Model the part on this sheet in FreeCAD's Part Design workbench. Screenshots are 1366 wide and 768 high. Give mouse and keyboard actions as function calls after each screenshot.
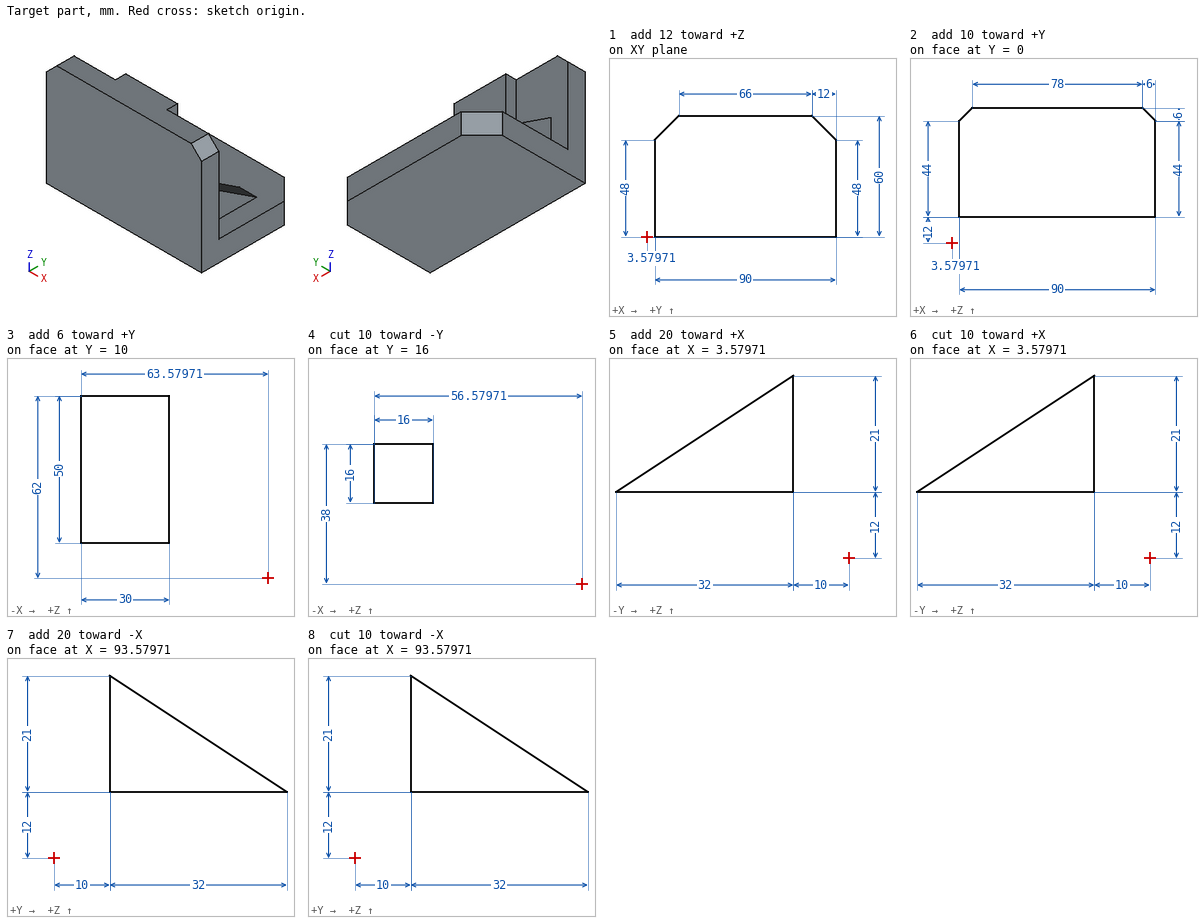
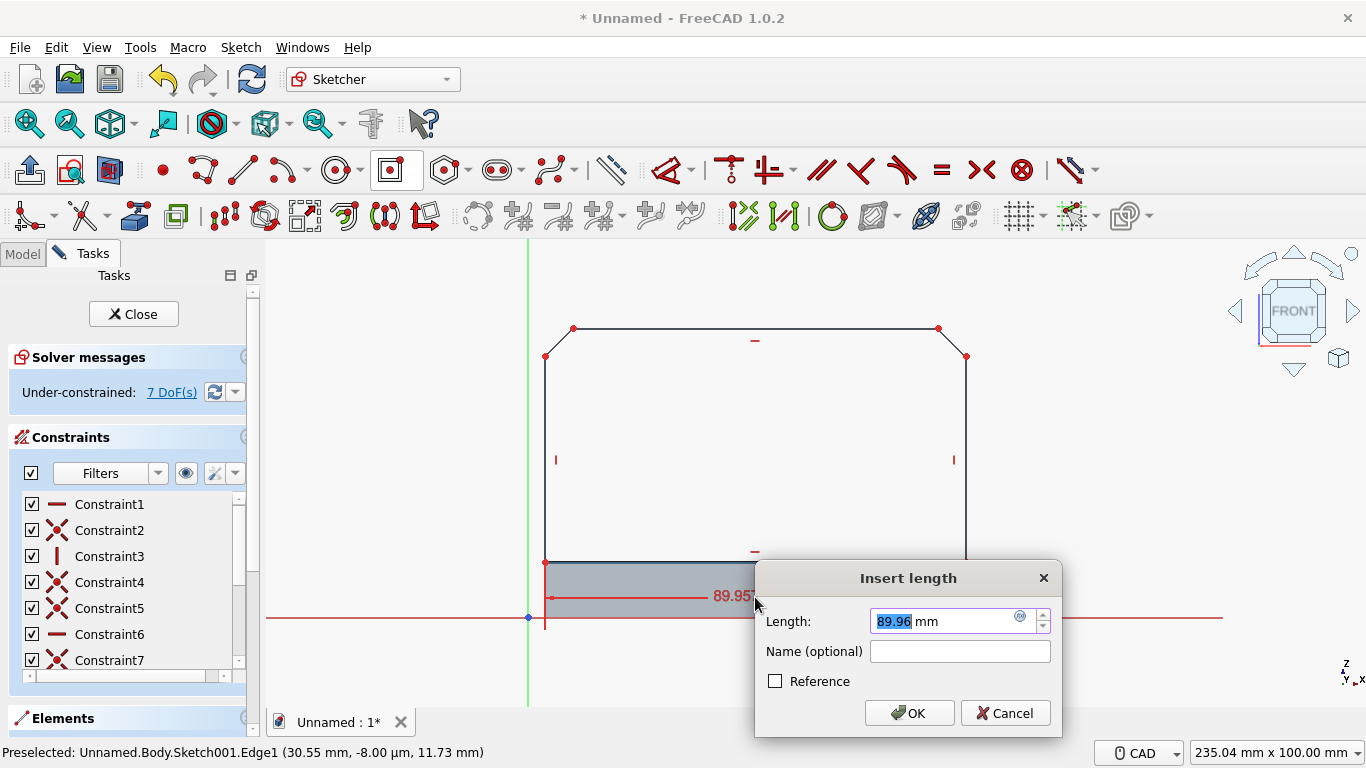
text(90)
key(Return)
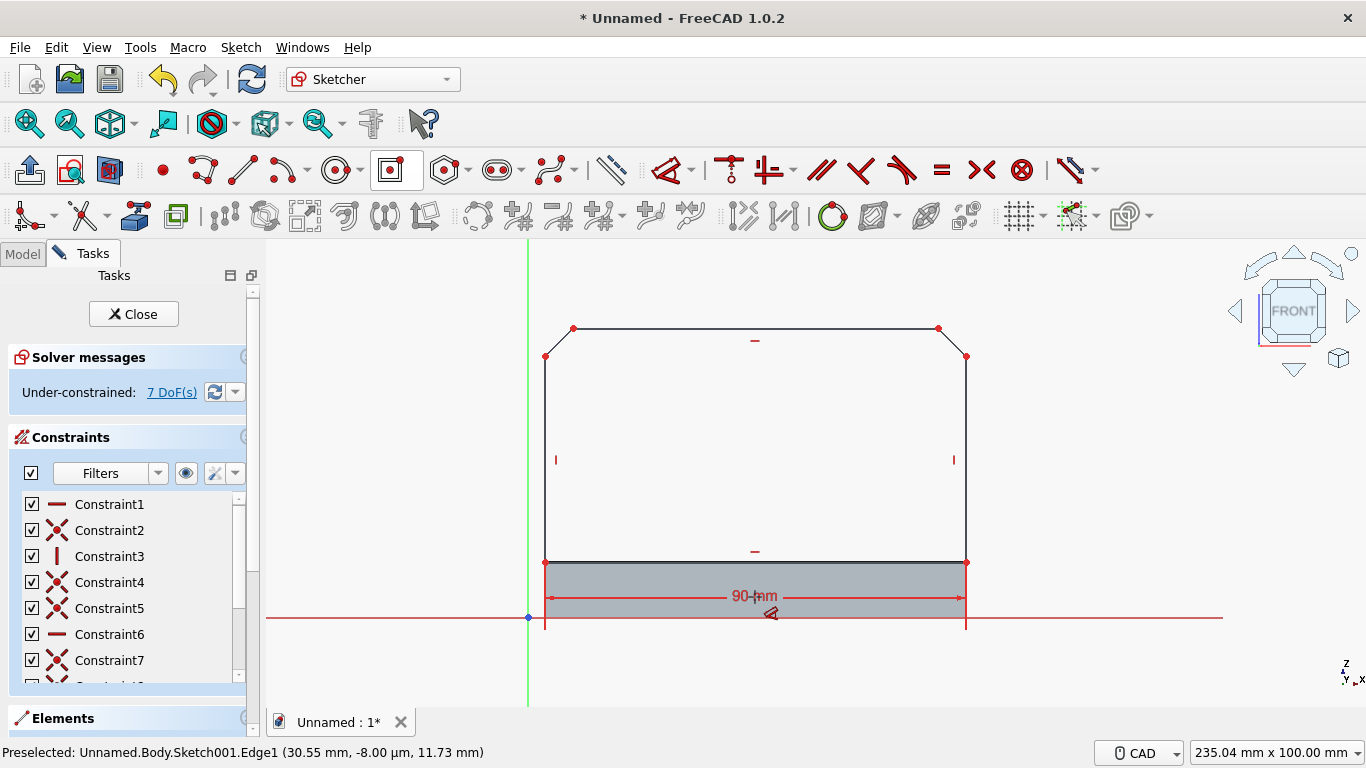
click(966, 501)
click(1000, 460)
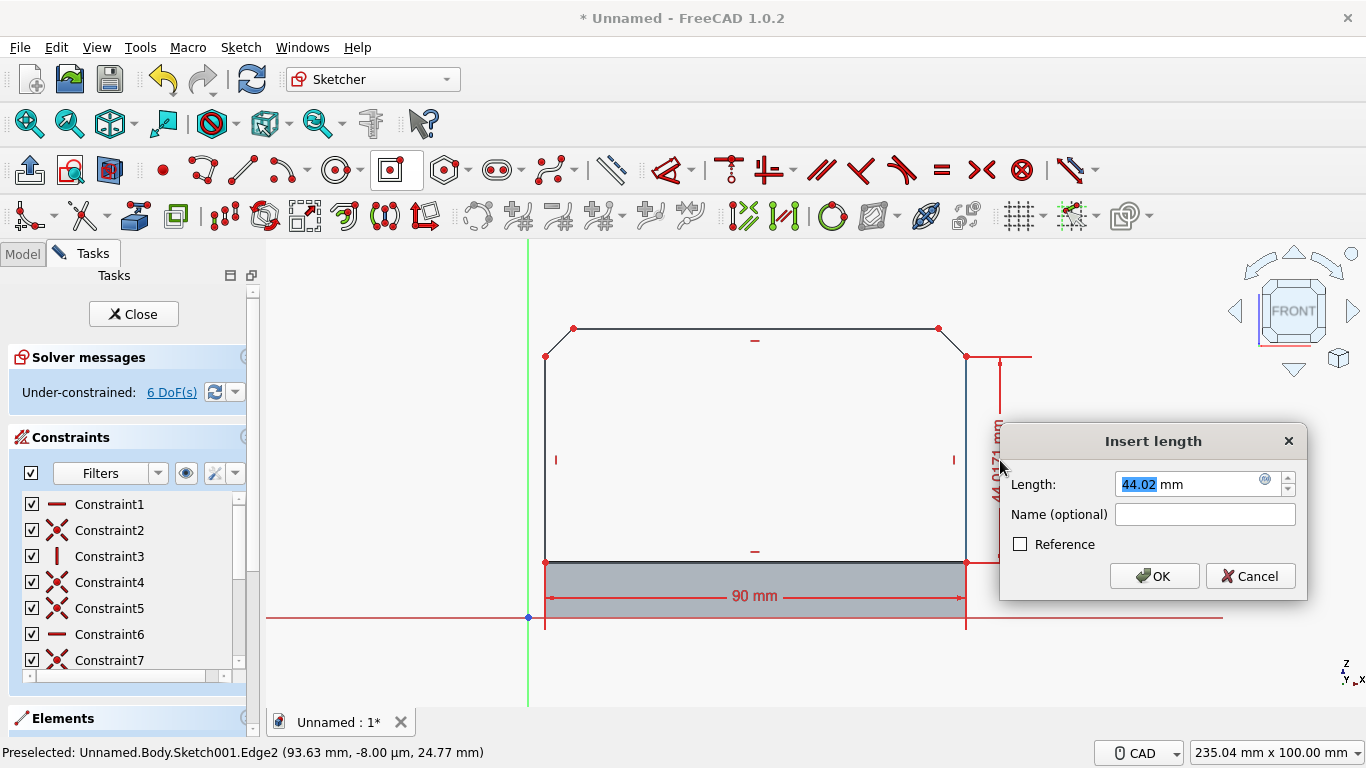
text(44)
key(Return)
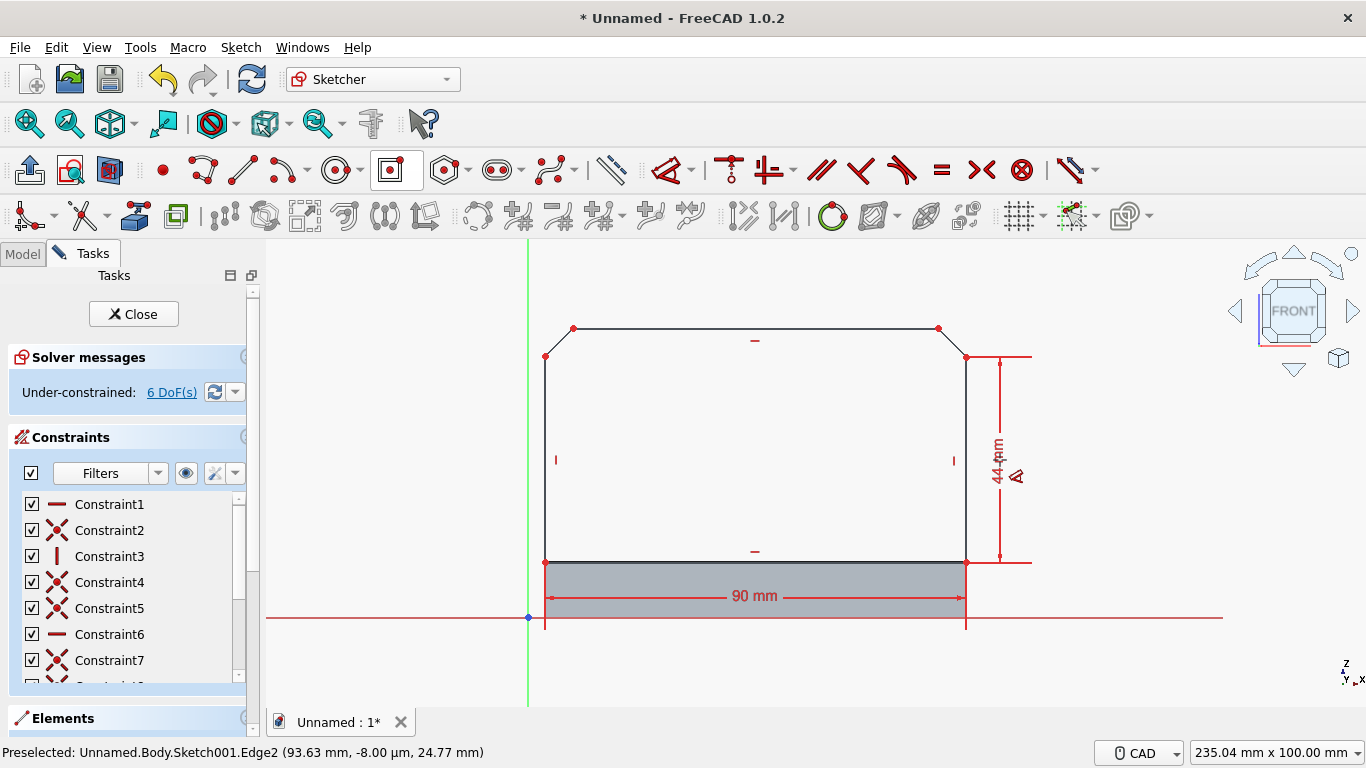
click(828, 329)
click(755, 295)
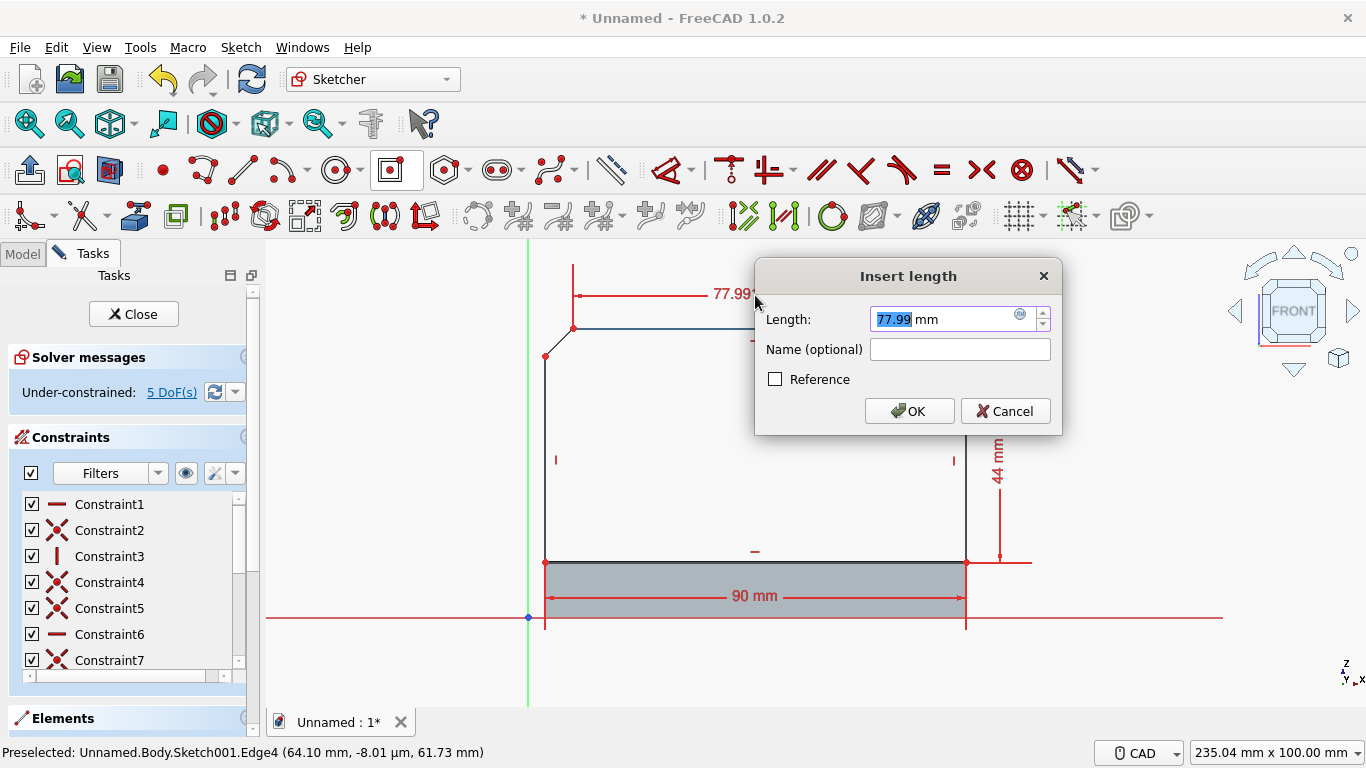
text(78)
key(Return)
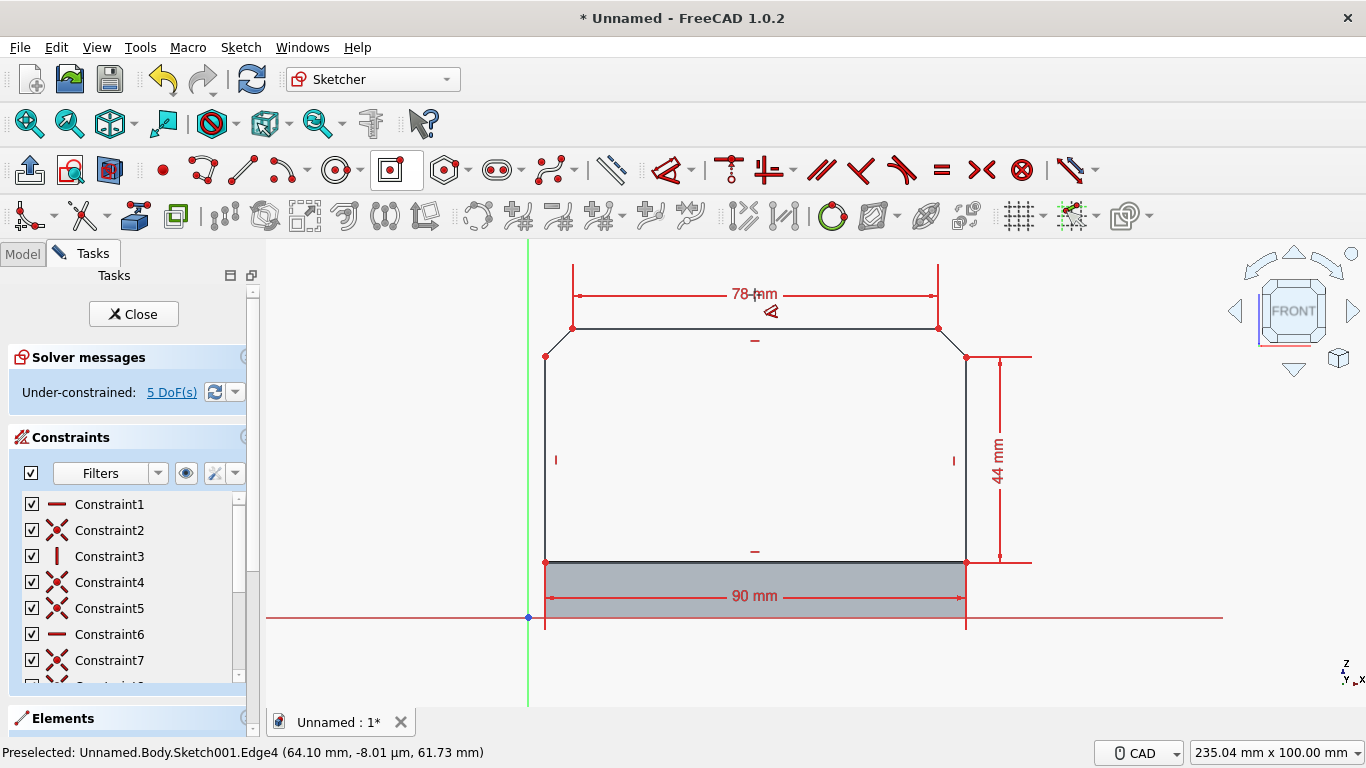
click(545, 419)
click(511, 460)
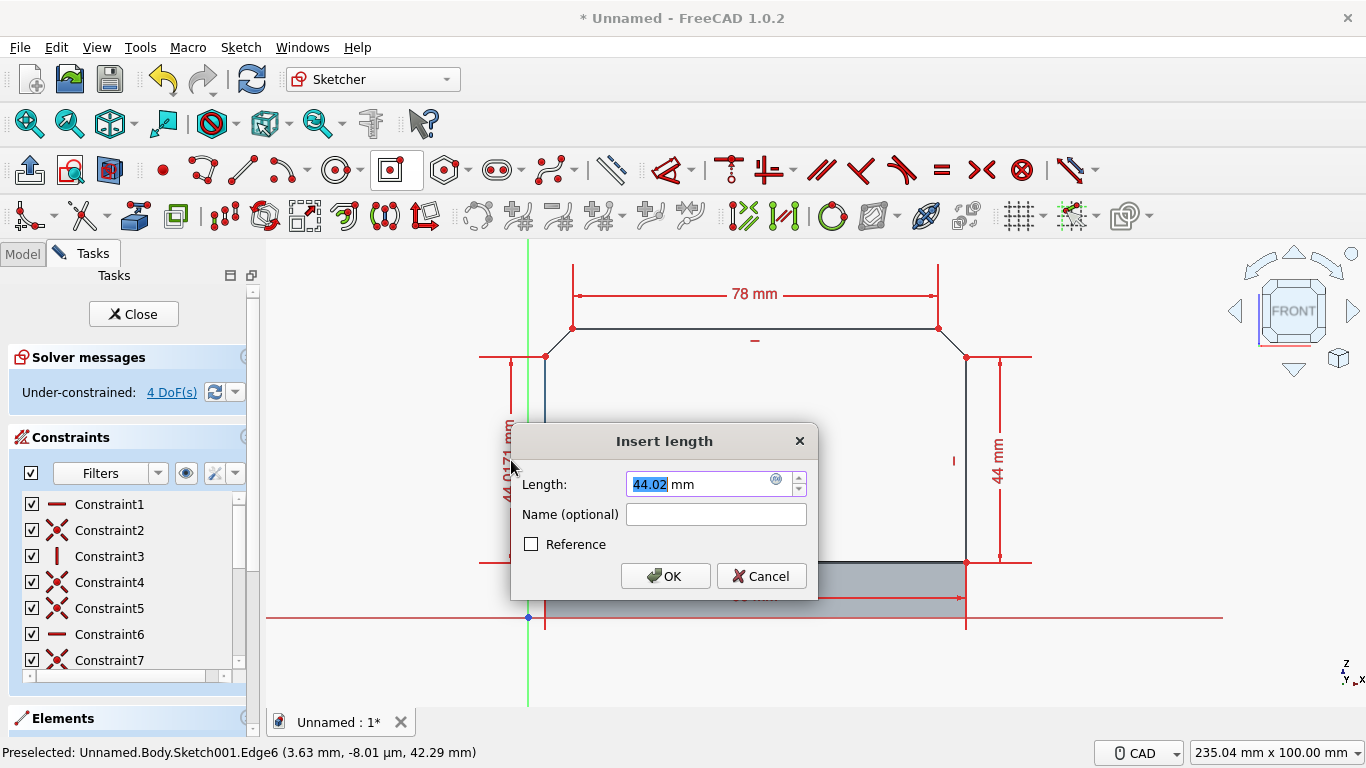
text(44)
key(Return)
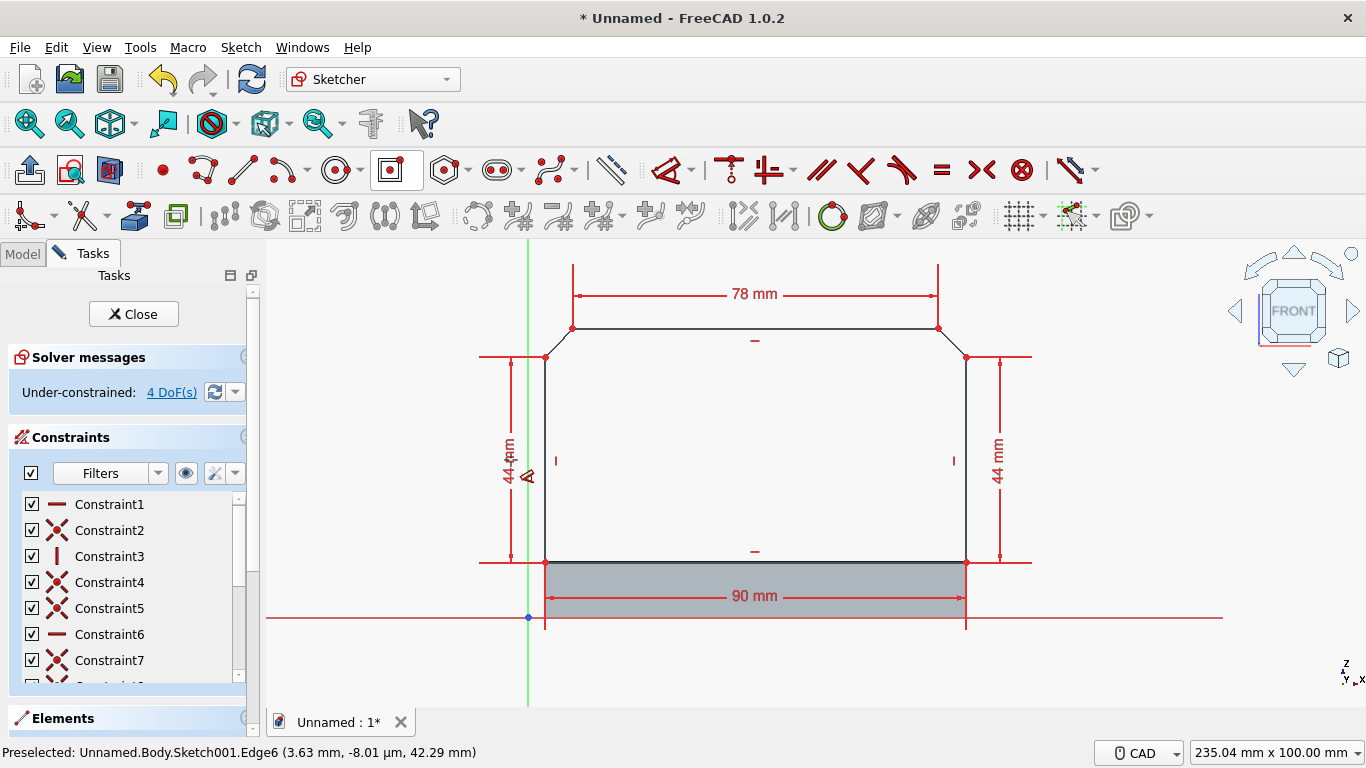
scroll(958, 349, up, 2)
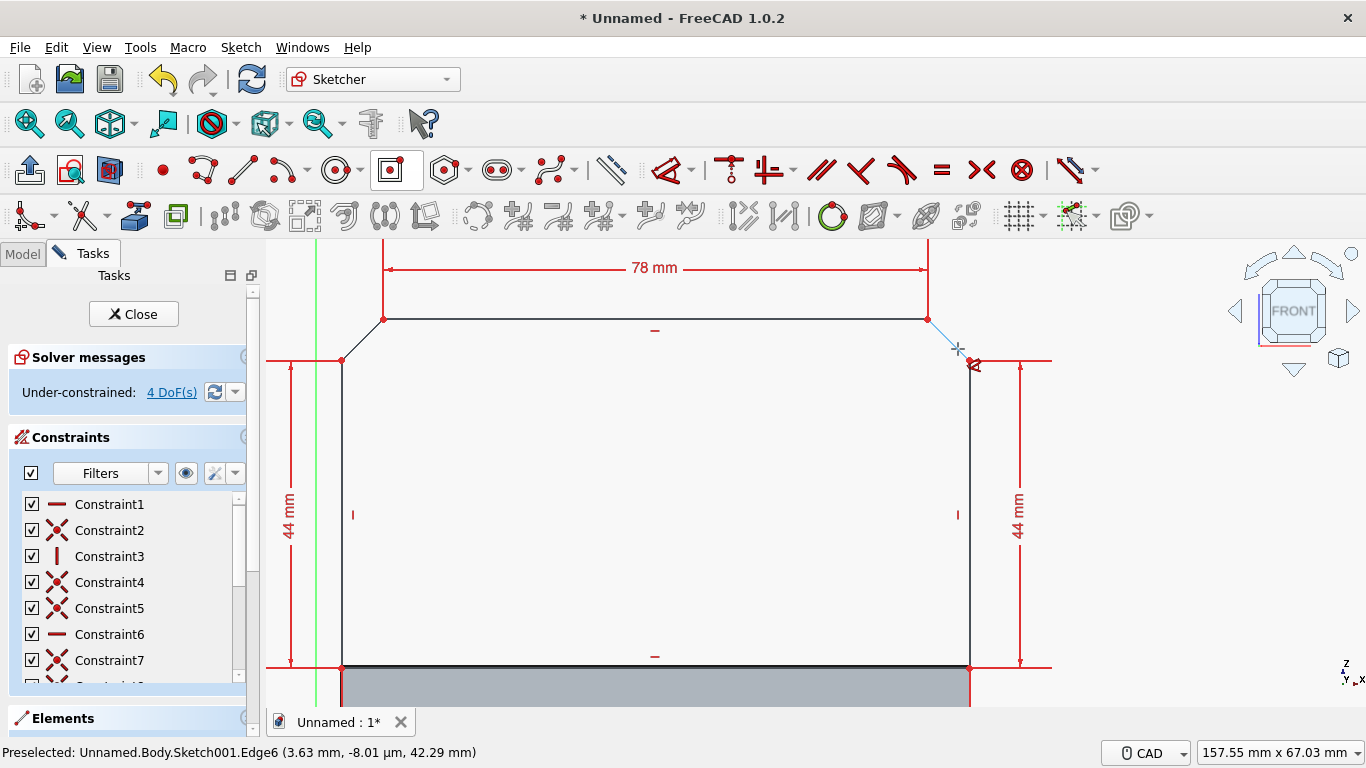
click(957, 348)
click(949, 285)